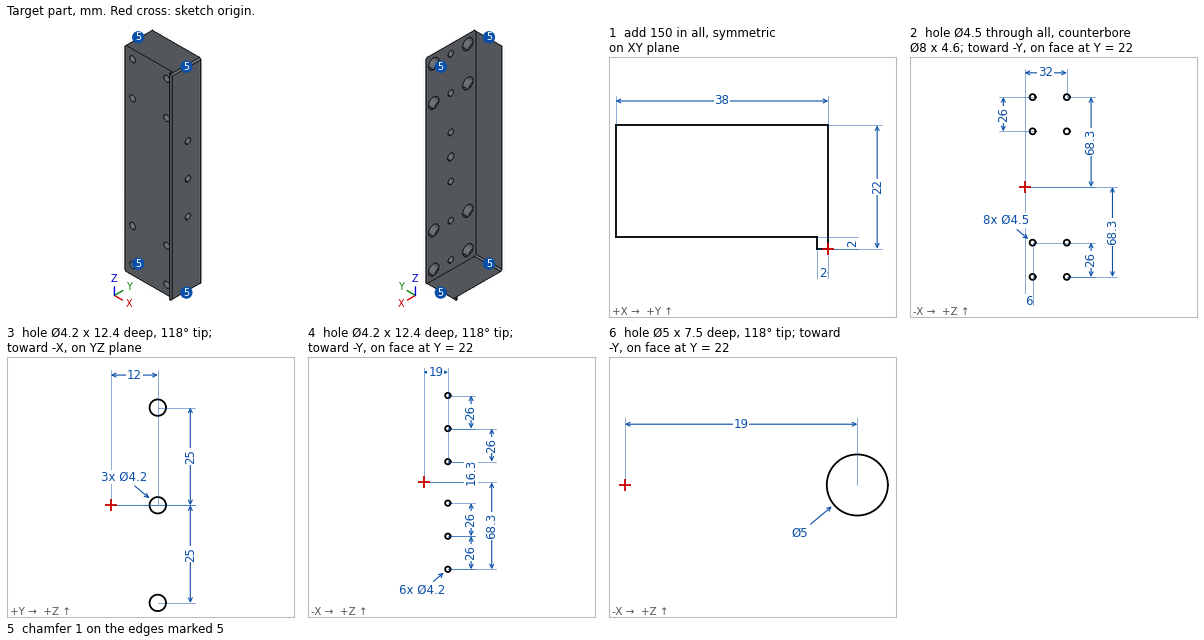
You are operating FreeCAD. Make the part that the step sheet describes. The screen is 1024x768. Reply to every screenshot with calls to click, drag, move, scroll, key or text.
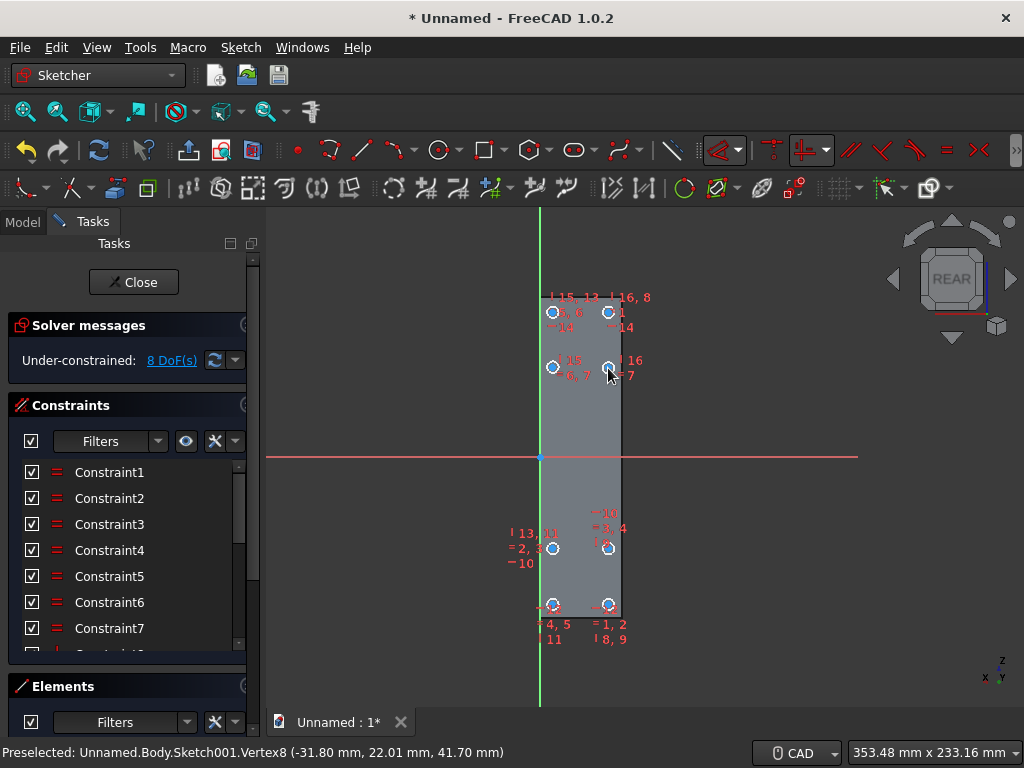
click(553, 367)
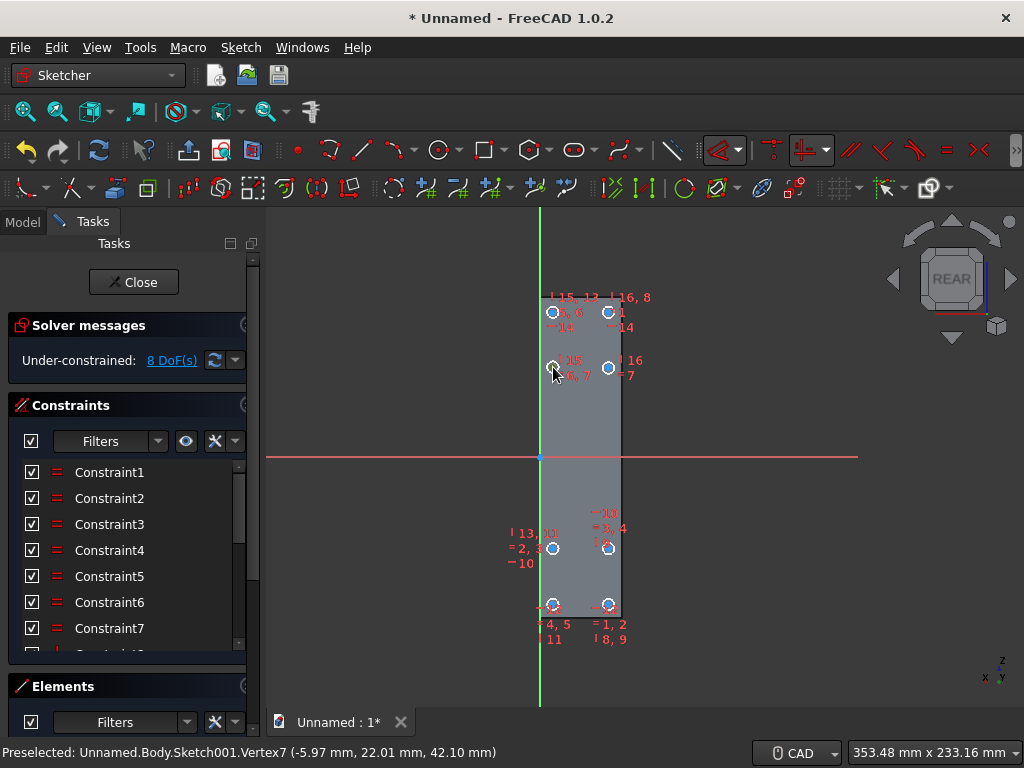
click(609, 368)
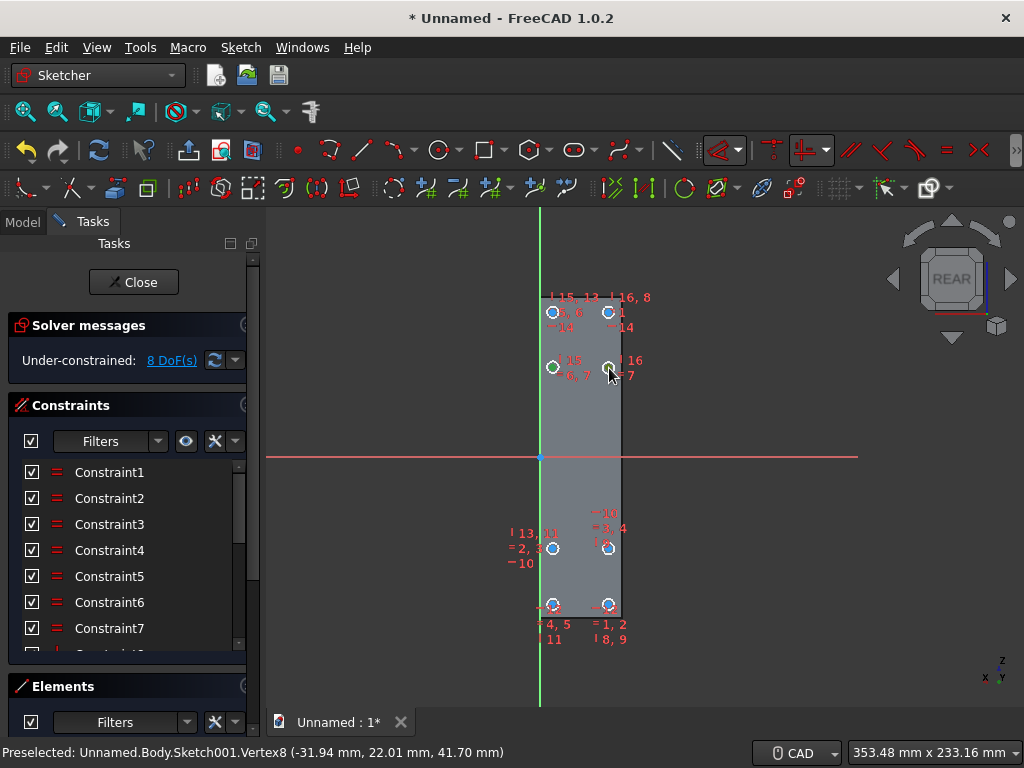
key(h)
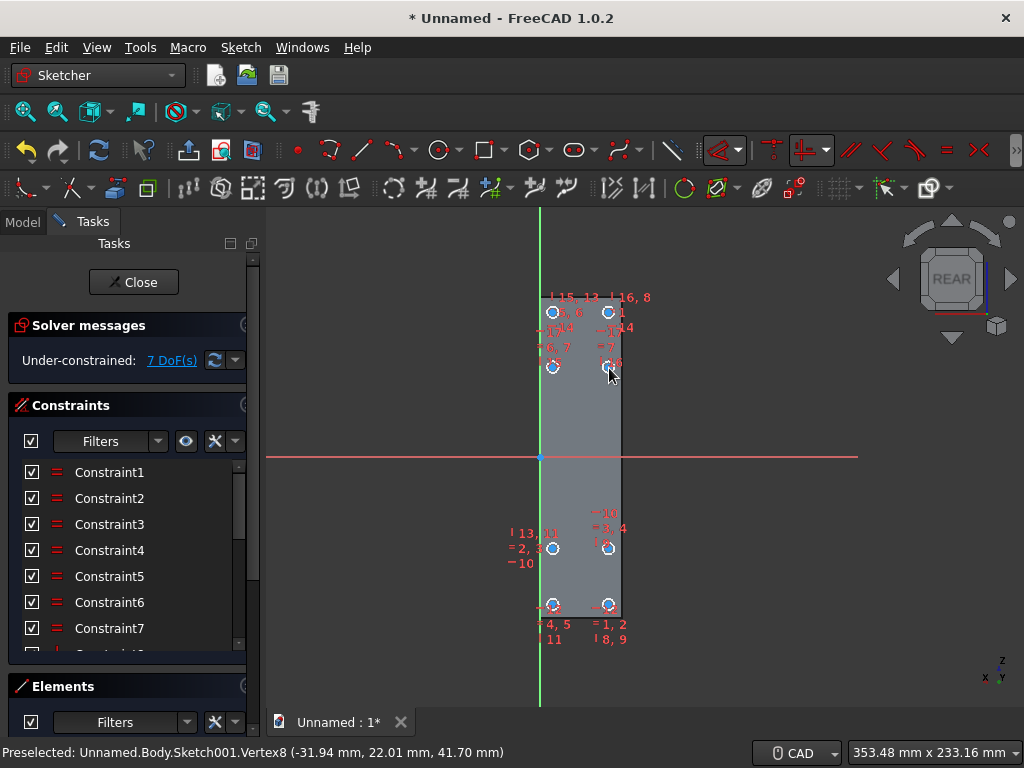
scroll(609, 307, up, 8)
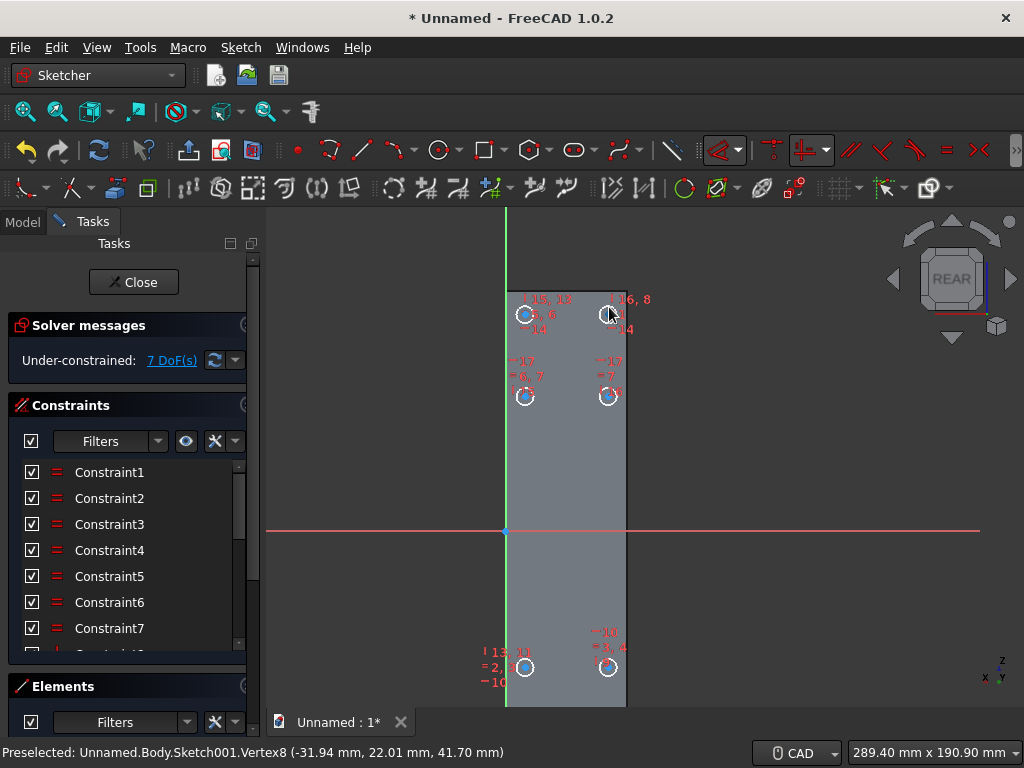
click(606, 304)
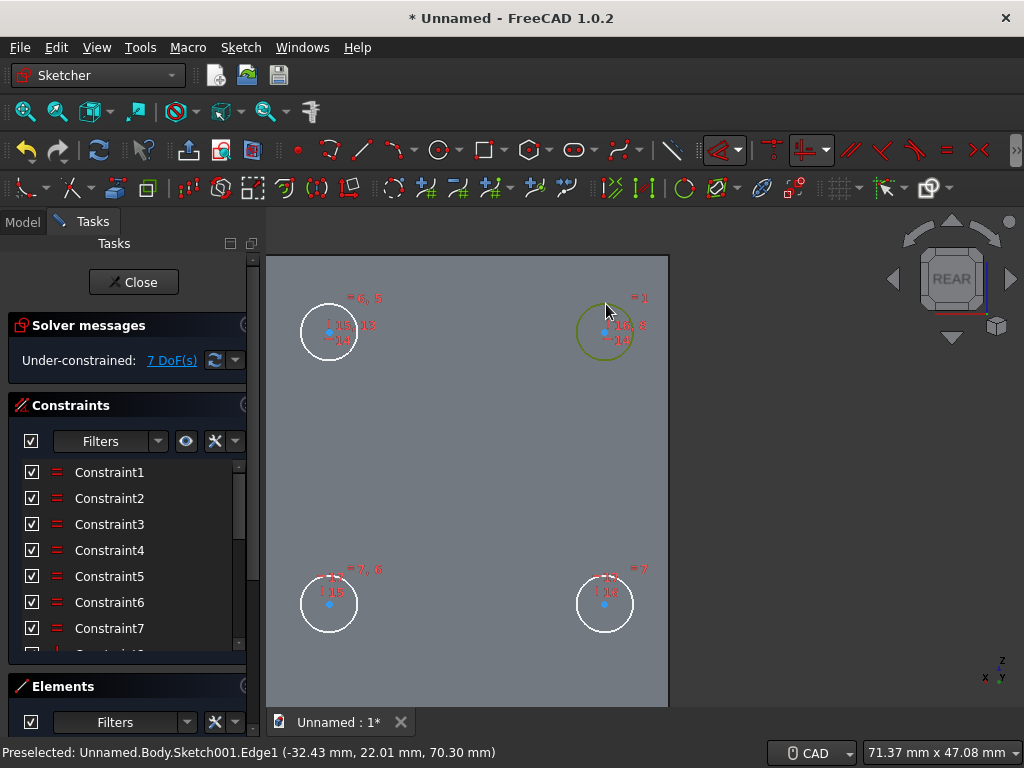
key(k)
key(o)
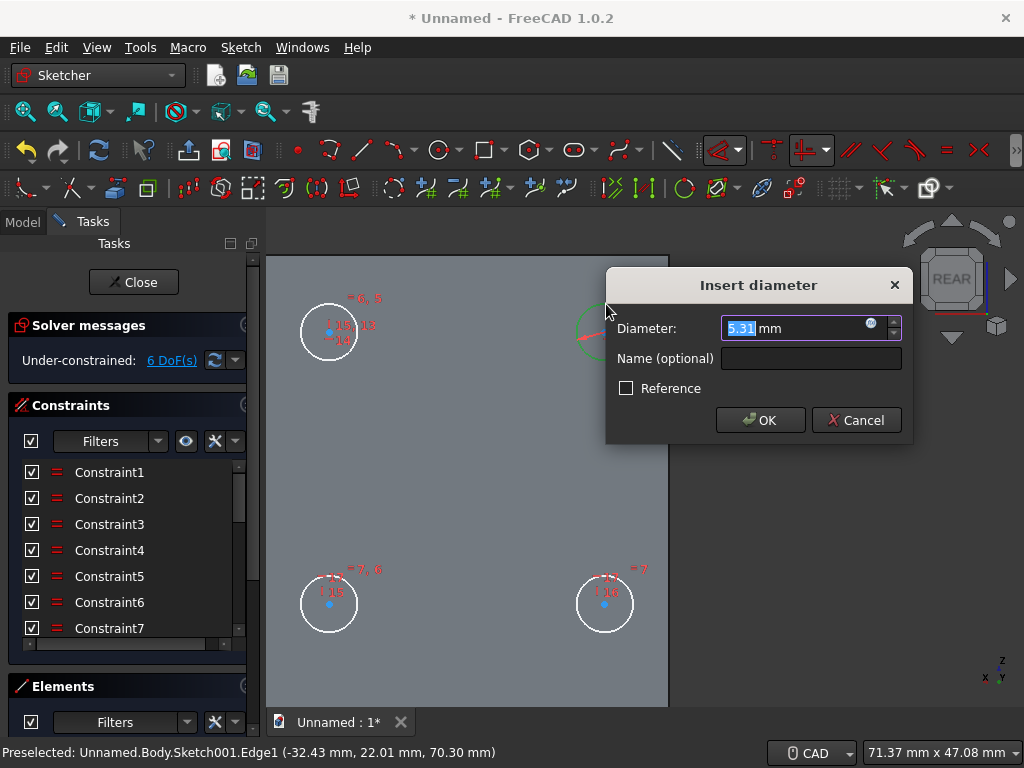
text(4.5)
key(Return)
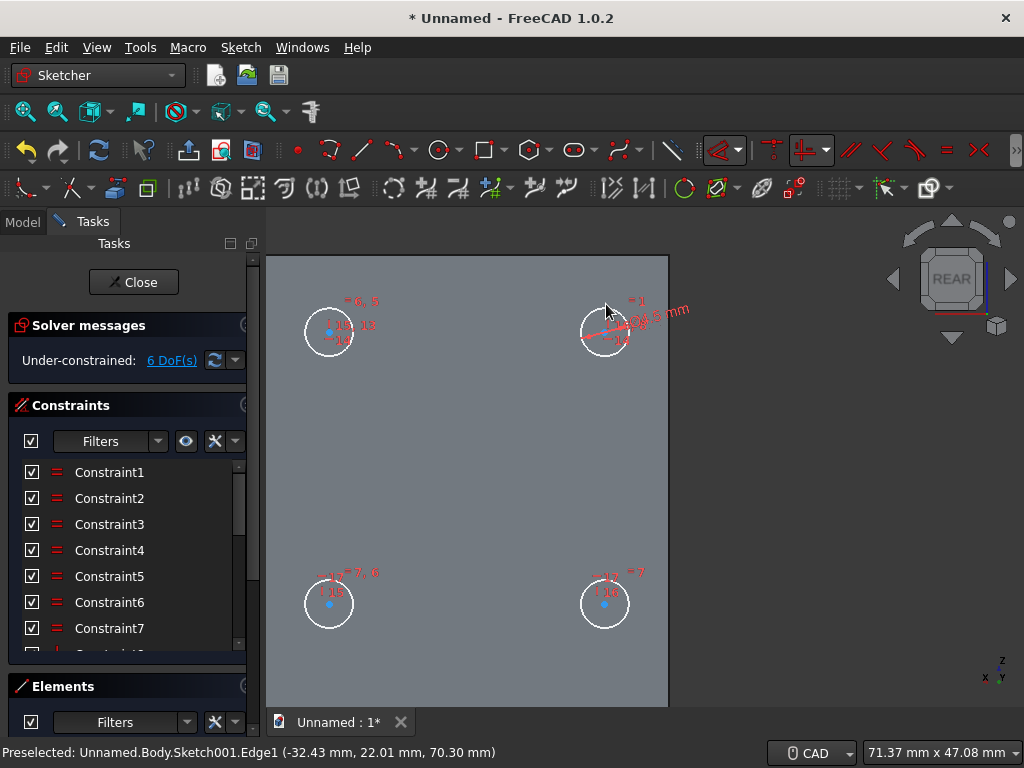
scroll(609, 307, down, 8)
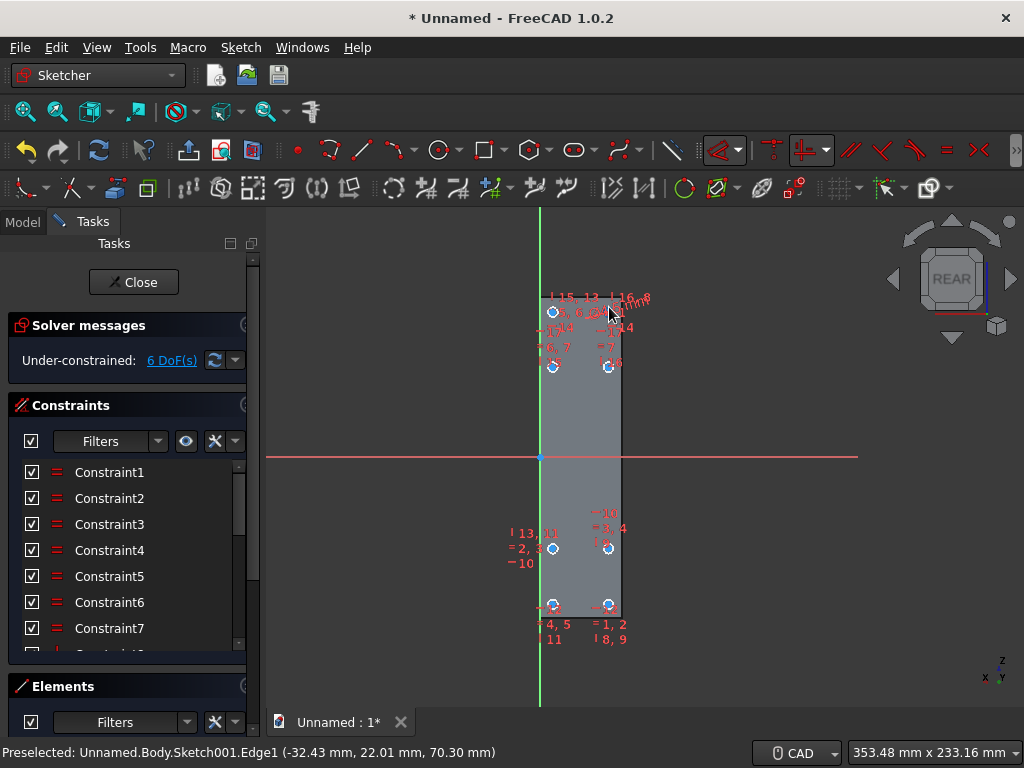
scroll(553, 549, up, 6)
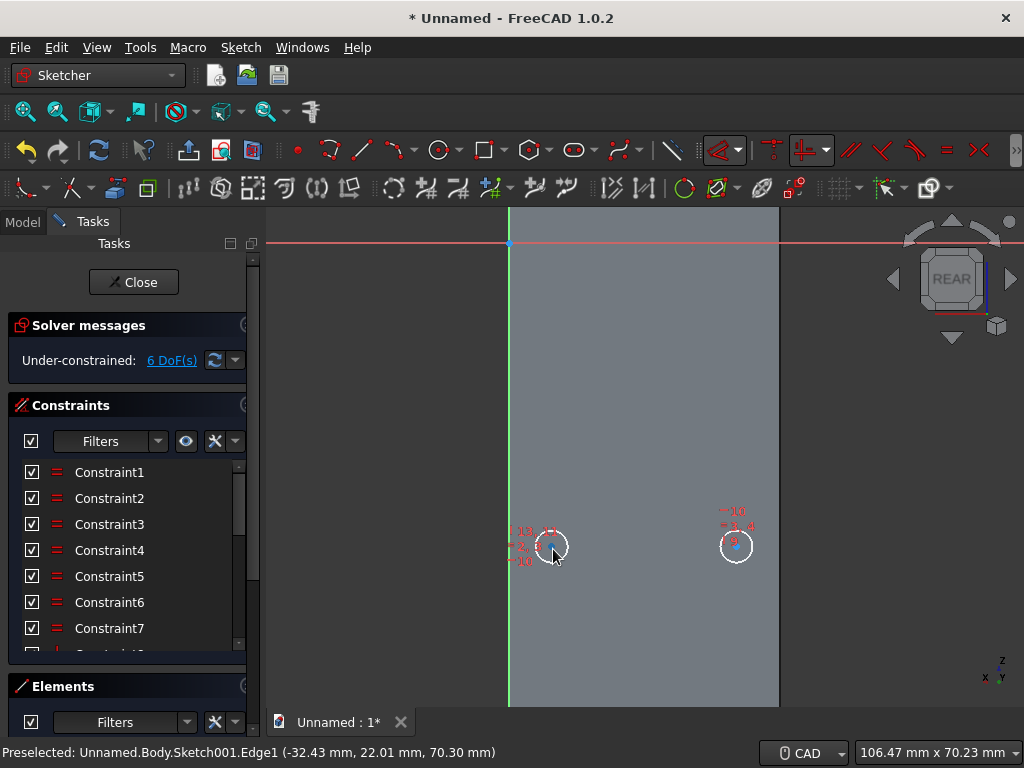
click(552, 547)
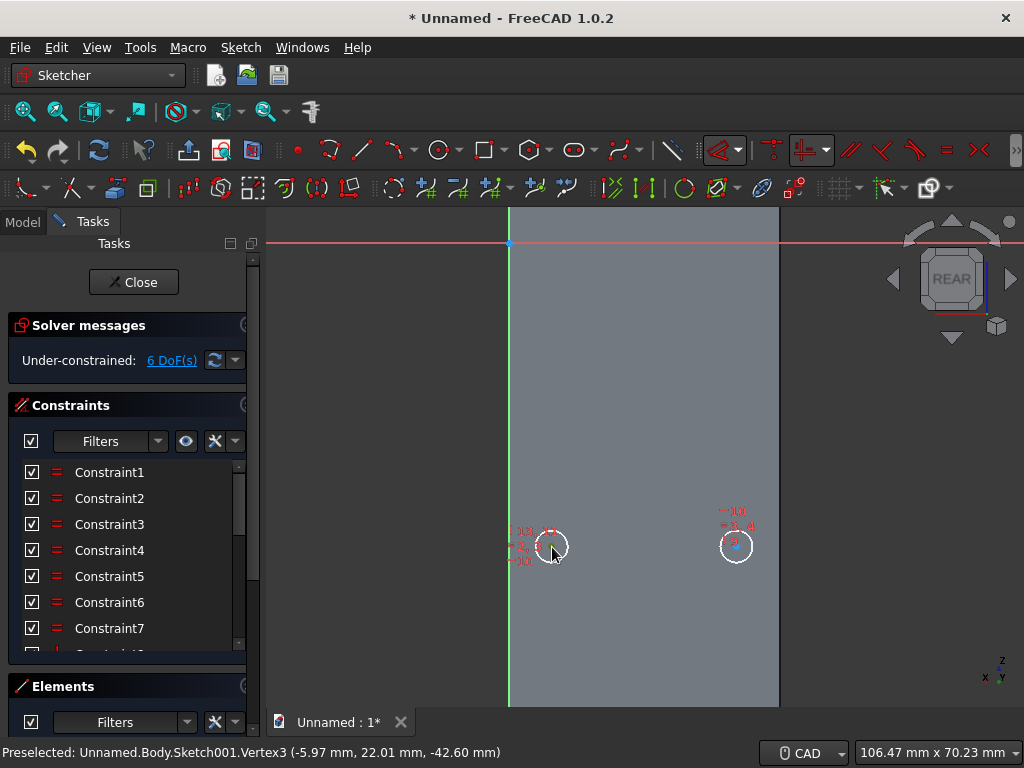
key(l)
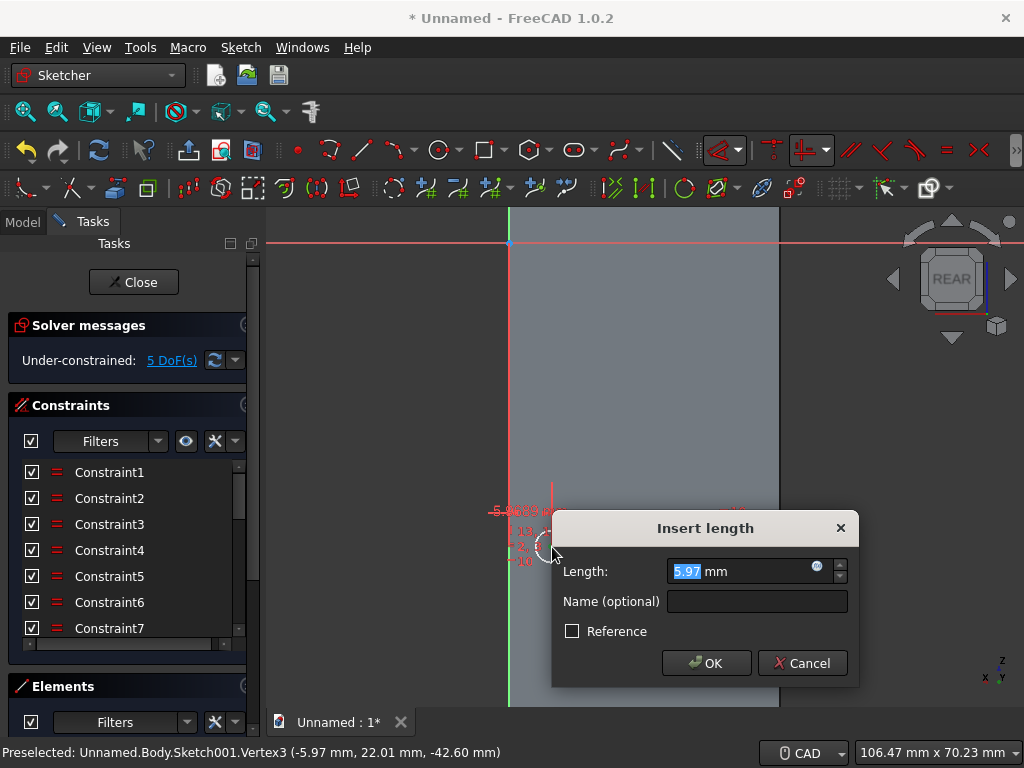
text(6)
key(Return)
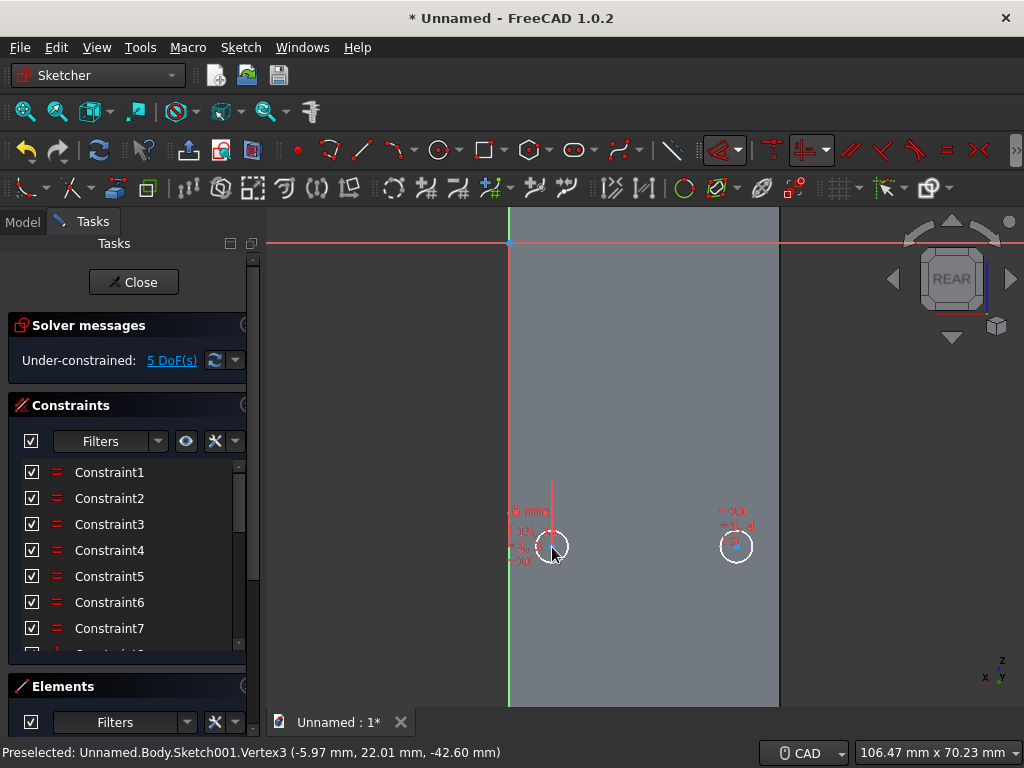
scroll(553, 549, down, 6)